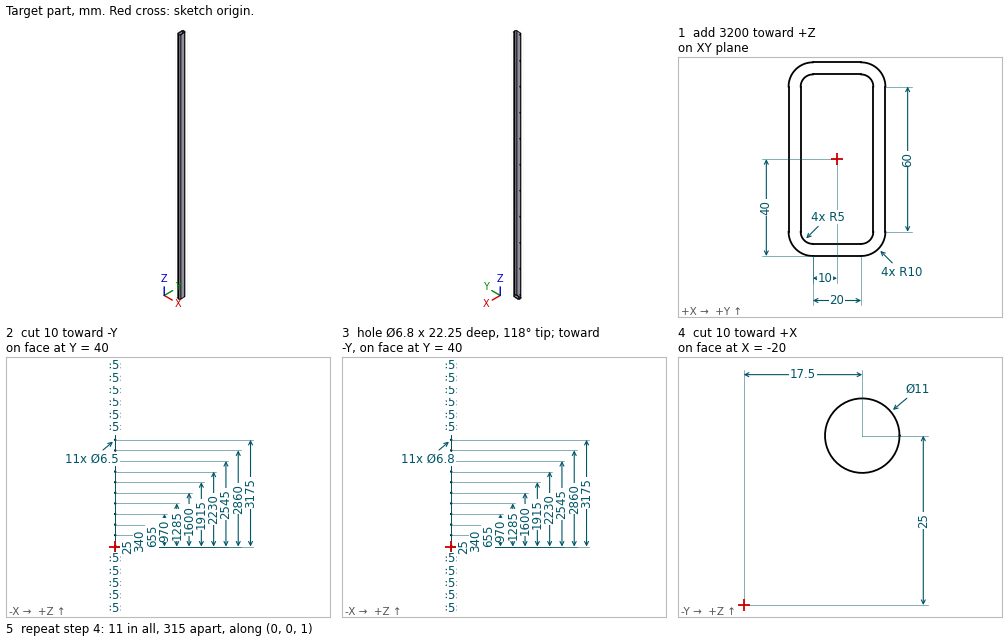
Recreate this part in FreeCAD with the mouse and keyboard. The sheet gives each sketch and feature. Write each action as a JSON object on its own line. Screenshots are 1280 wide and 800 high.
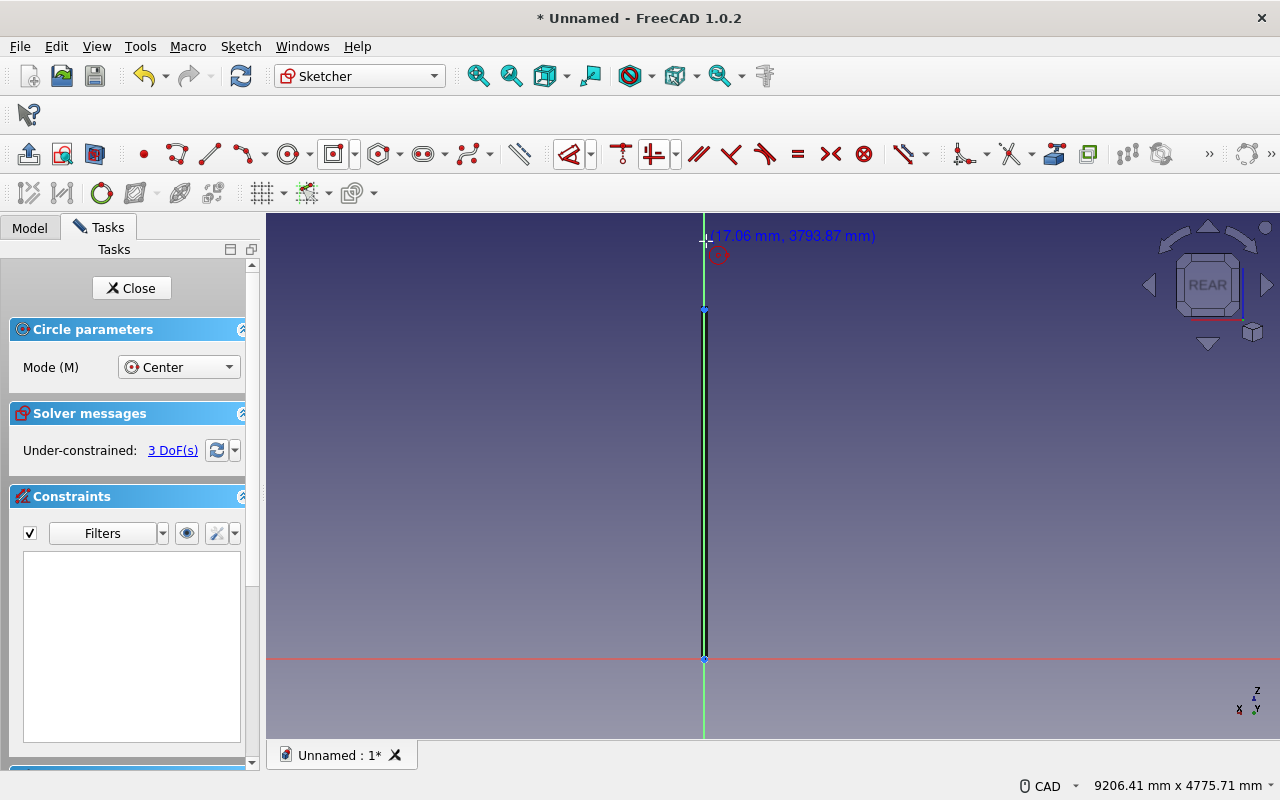
{"action": "scroll", "coordinate": [705, 344], "scroll_direction": "up", "scroll_amount": 21}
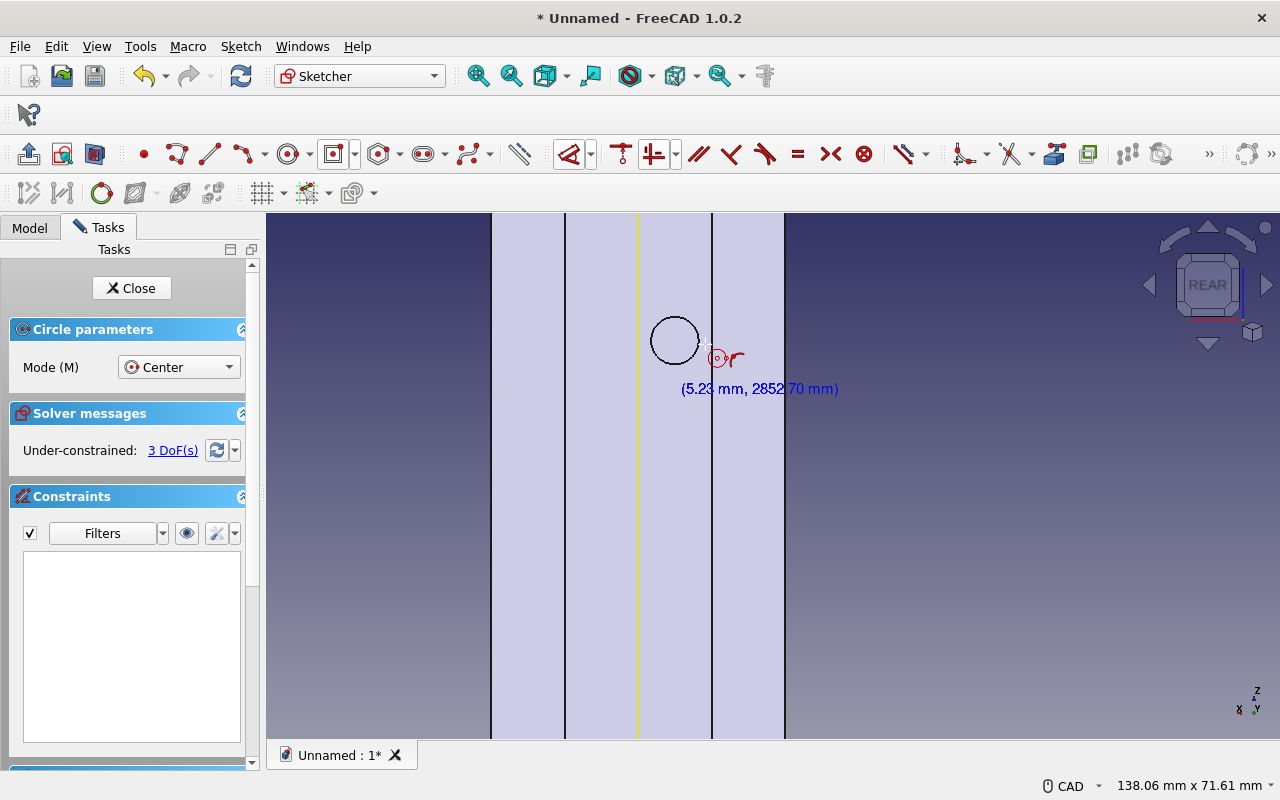
{"action": "left_click", "coordinate": [675, 341]}
{"action": "left_click", "coordinate": [693, 323]}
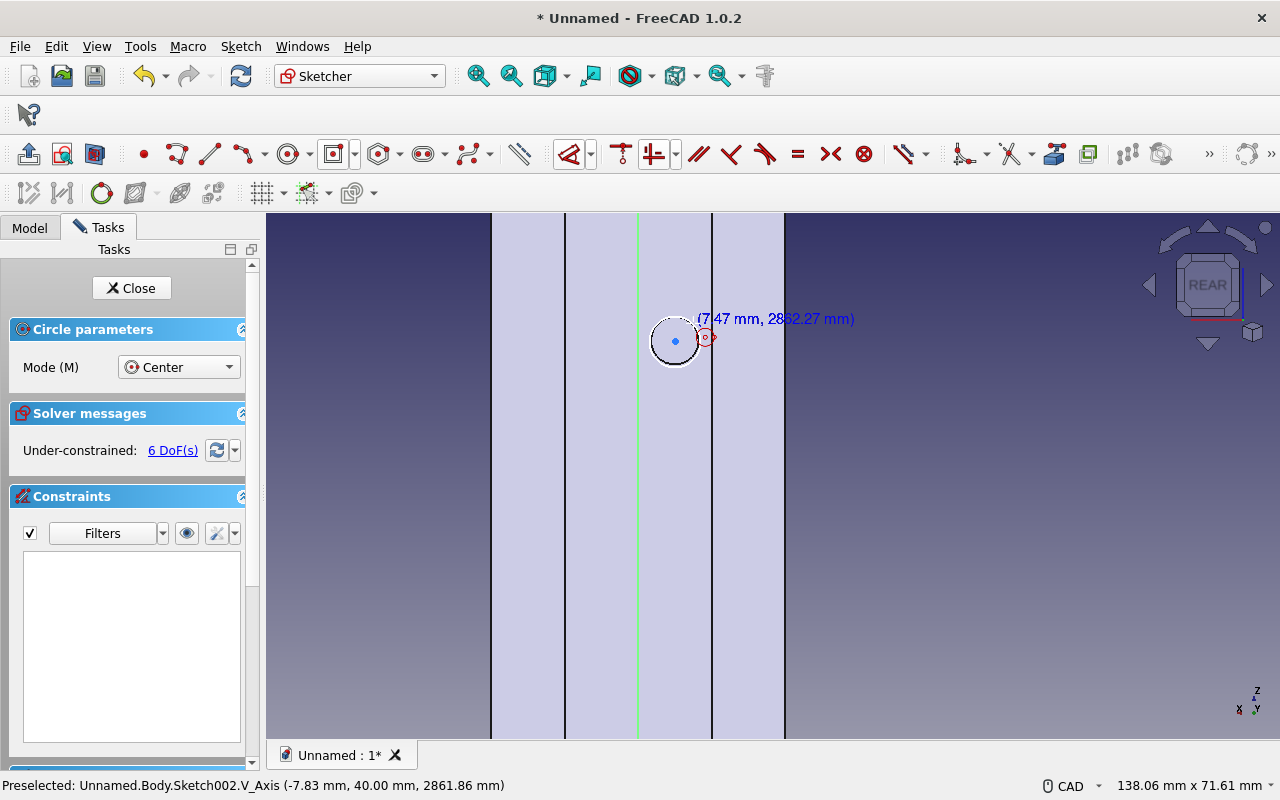
{"action": "scroll", "coordinate": [704, 476], "scroll_direction": "down", "scroll_amount": 15}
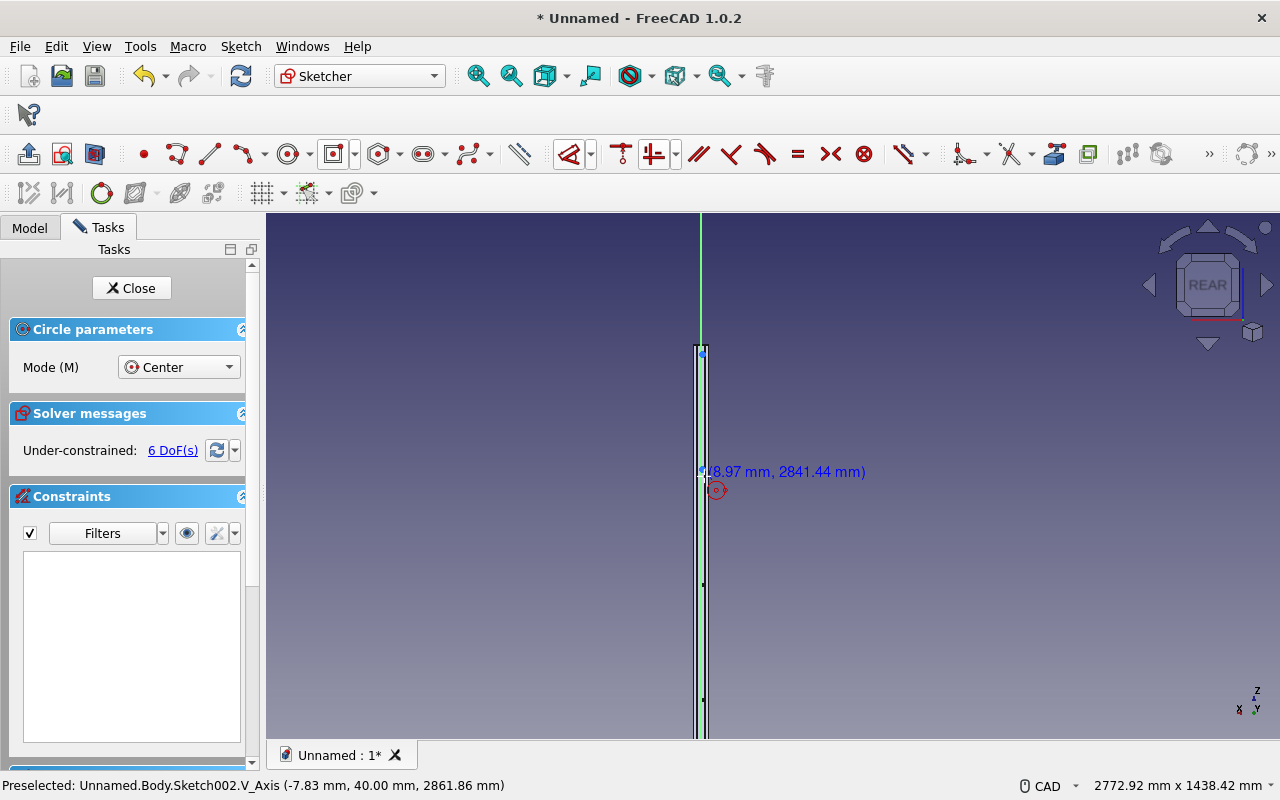
{"action": "scroll", "coordinate": [705, 278], "scroll_direction": "down", "scroll_amount": 6}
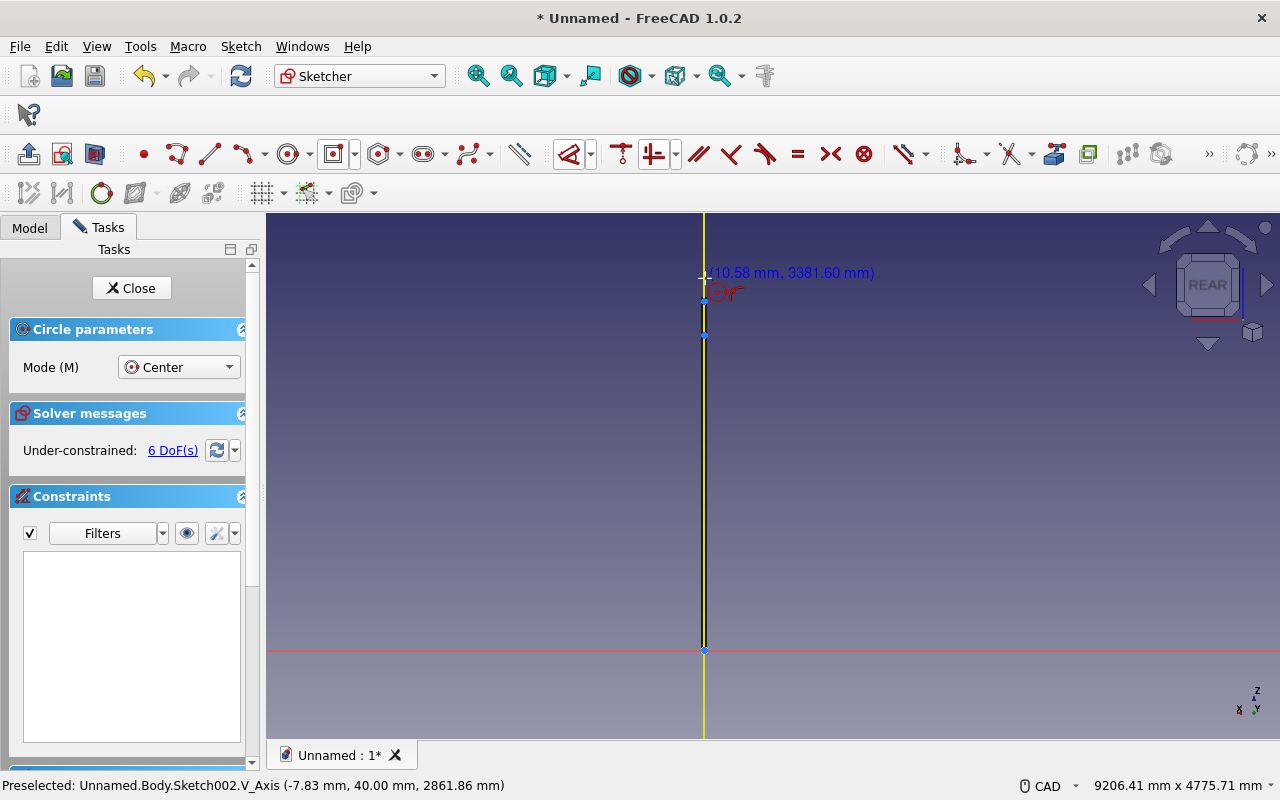
{"action": "scroll", "coordinate": [705, 371], "scroll_direction": "up", "scroll_amount": 21}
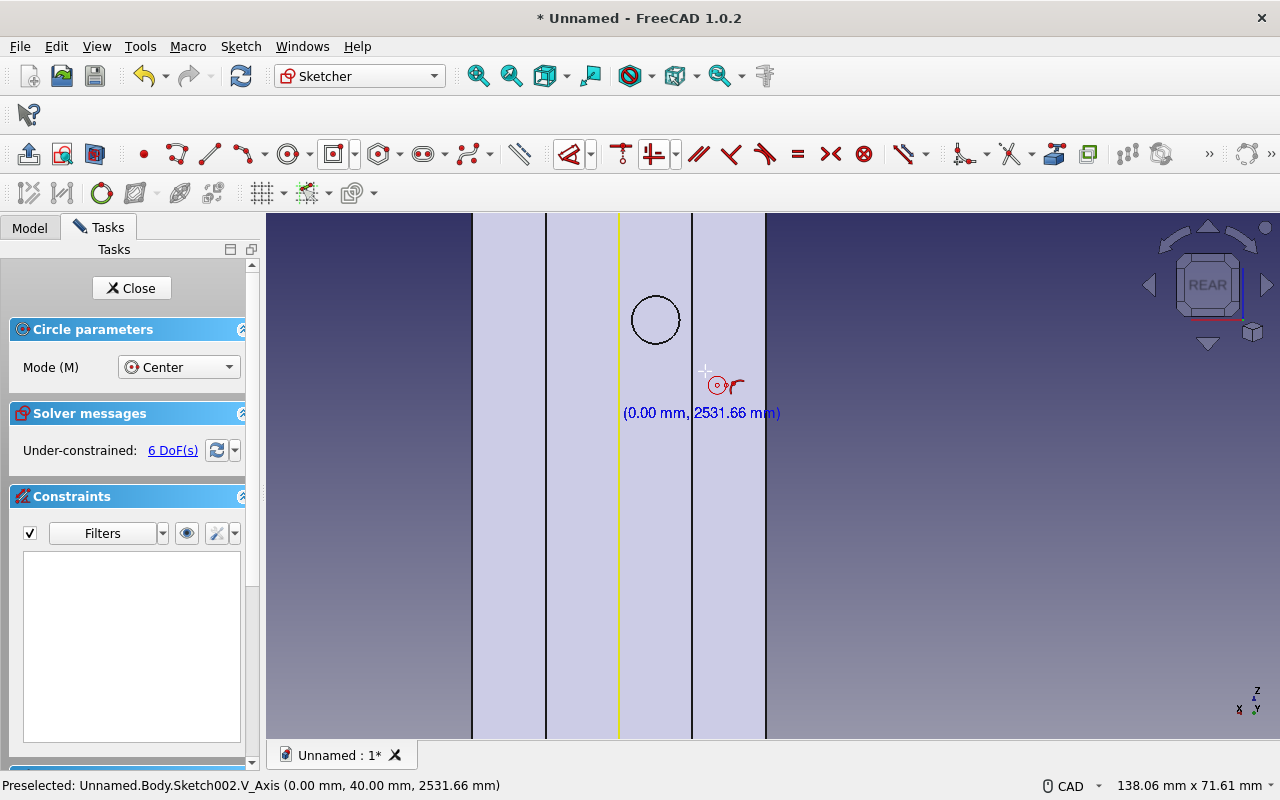
{"action": "left_click", "coordinate": [656, 320]}
{"action": "left_click", "coordinate": [673, 302]}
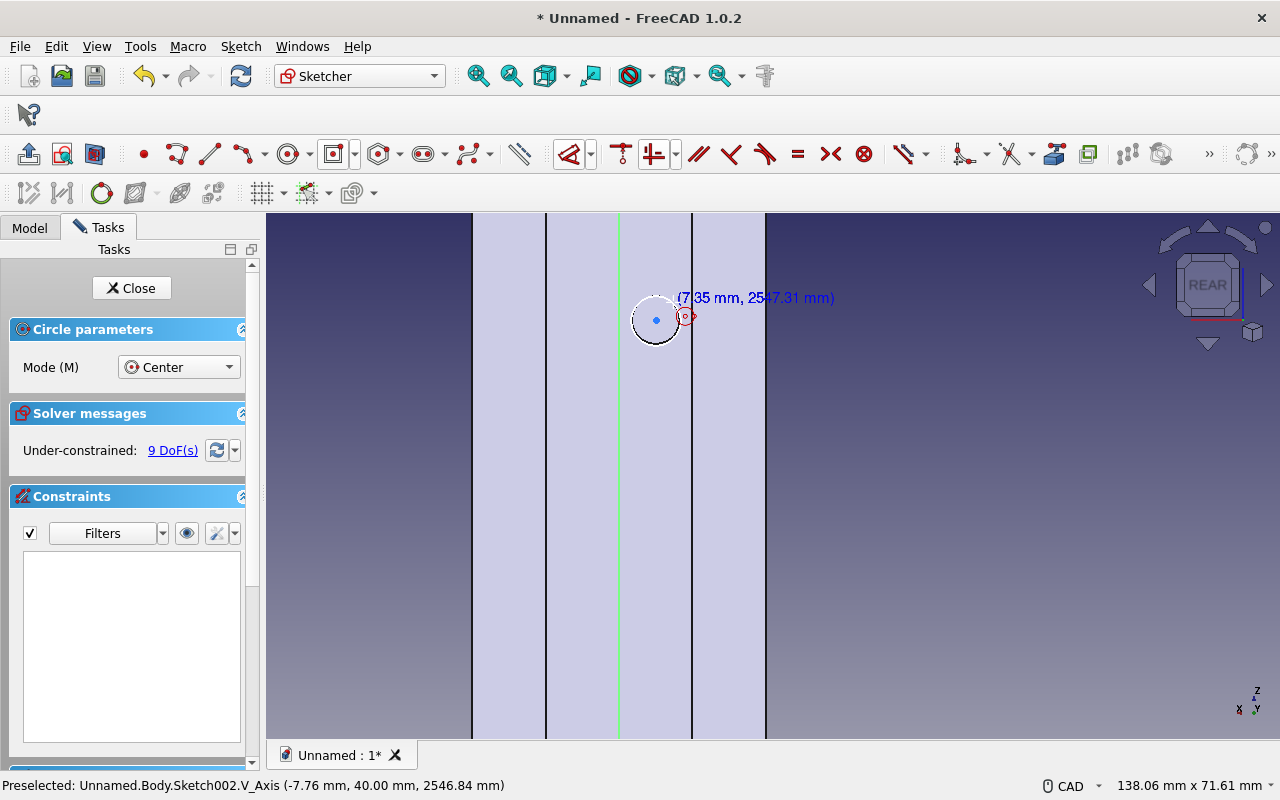
{"action": "scroll", "coordinate": [704, 476], "scroll_direction": "down", "scroll_amount": 15}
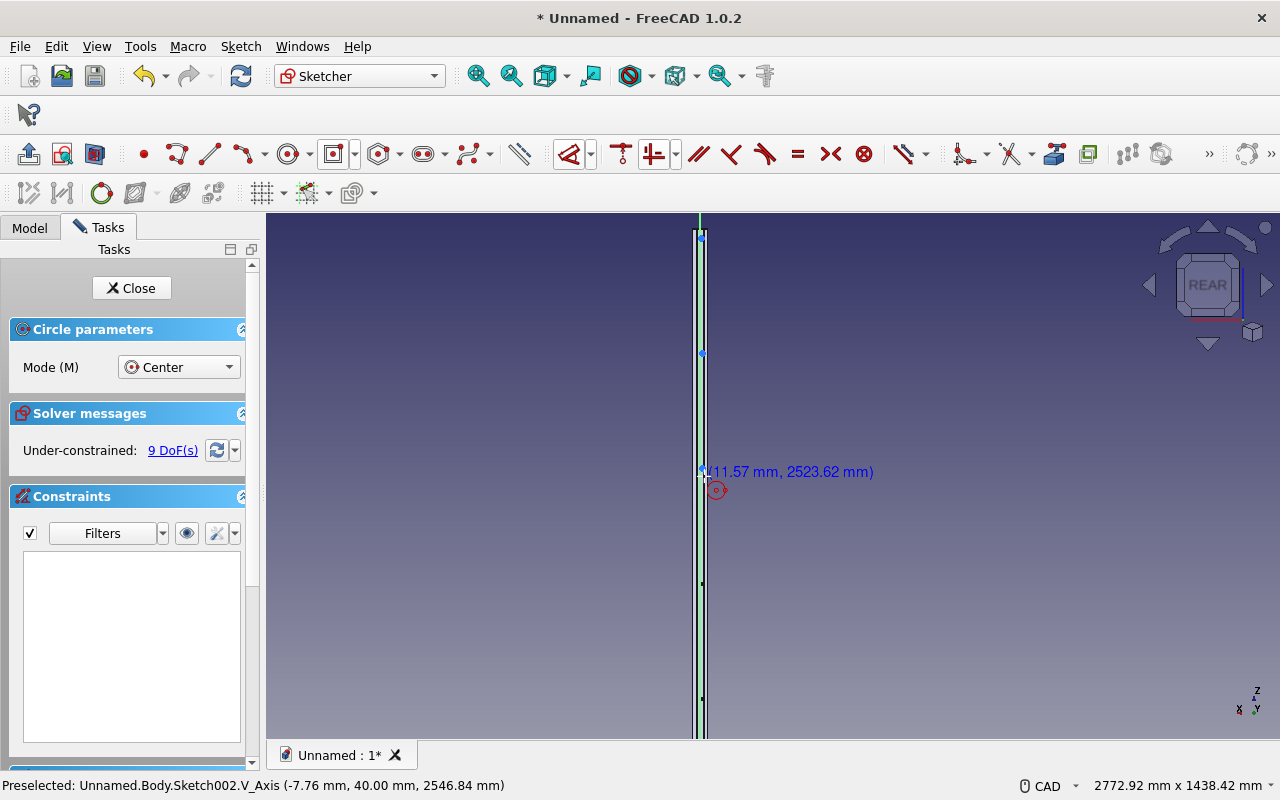
{"action": "scroll", "coordinate": [706, 328], "scroll_direction": "down", "scroll_amount": 6}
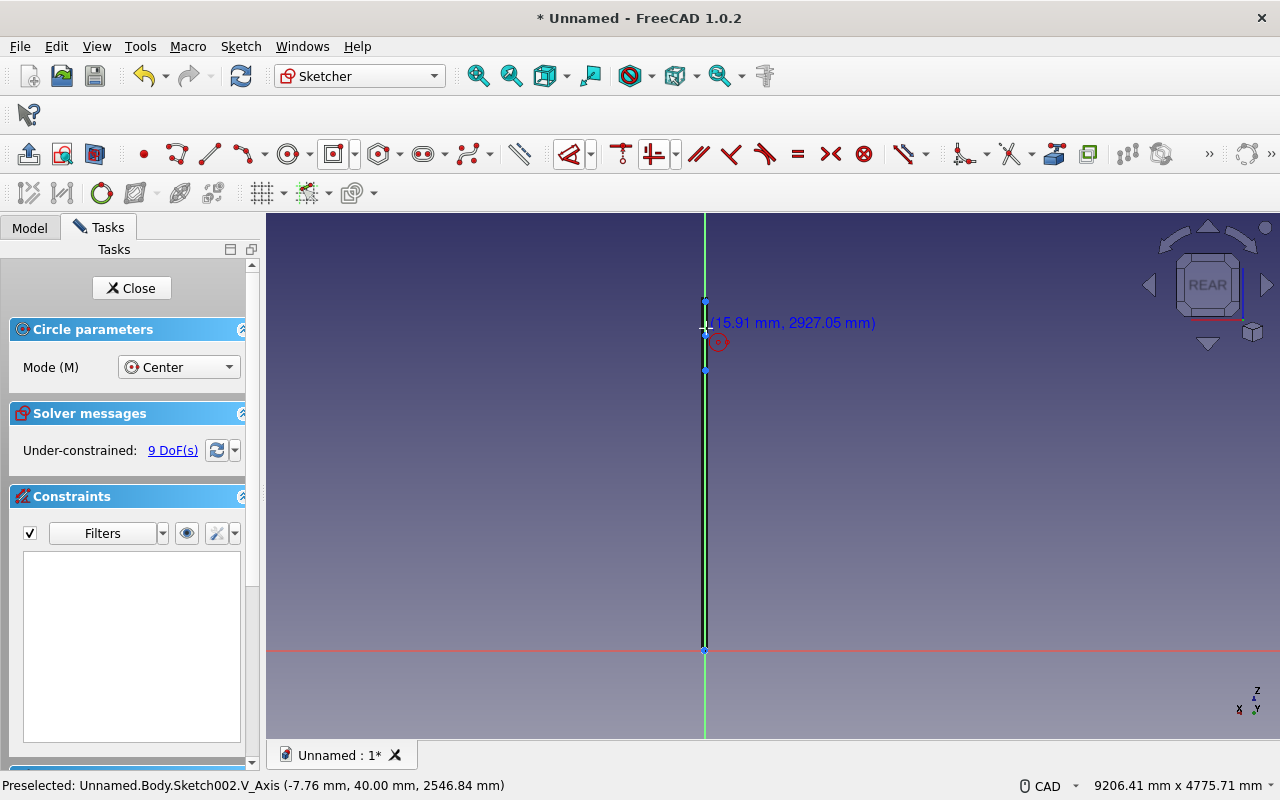
{"action": "scroll", "coordinate": [705, 405], "scroll_direction": "up", "scroll_amount": 21}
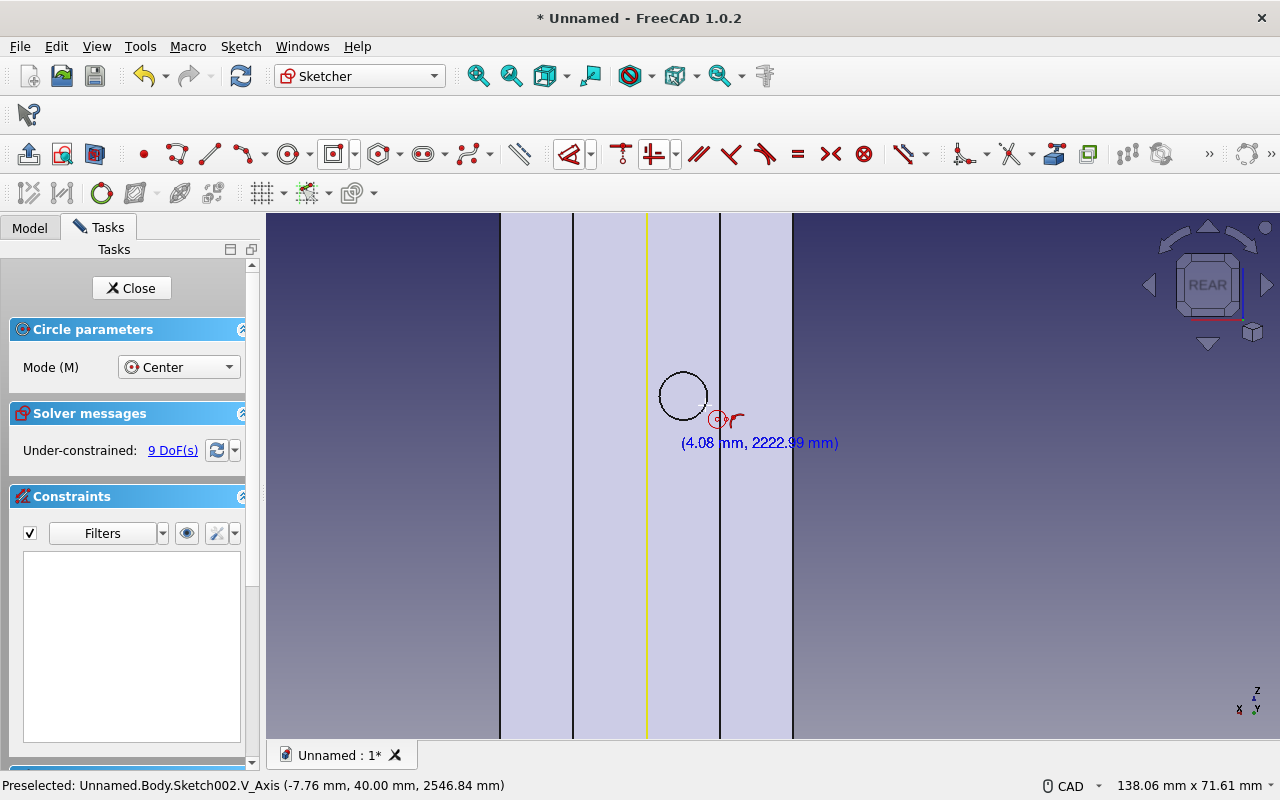
{"action": "left_click", "coordinate": [683, 396]}
{"action": "left_click", "coordinate": [701, 379]}